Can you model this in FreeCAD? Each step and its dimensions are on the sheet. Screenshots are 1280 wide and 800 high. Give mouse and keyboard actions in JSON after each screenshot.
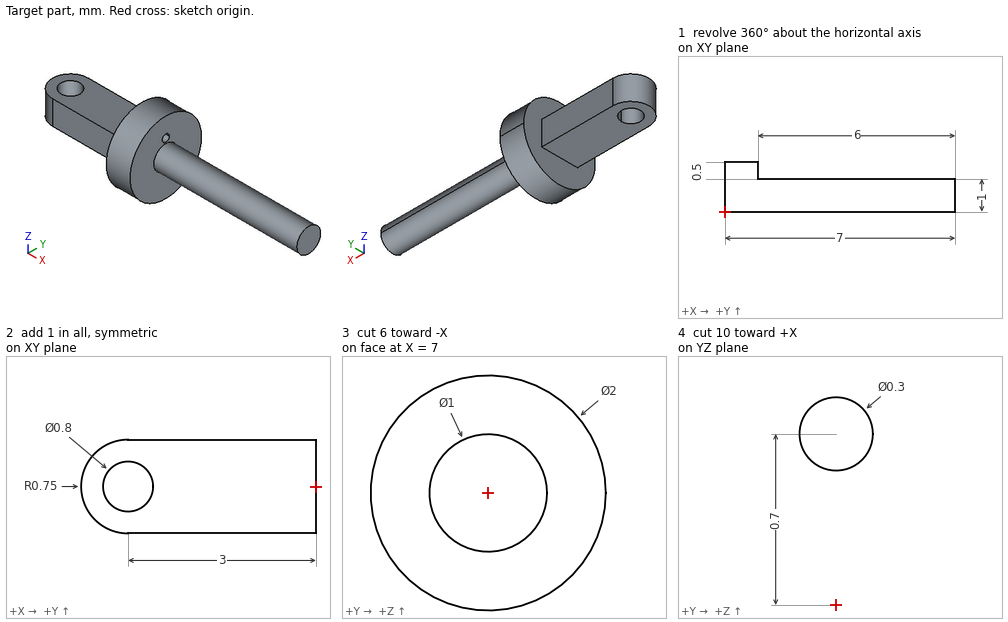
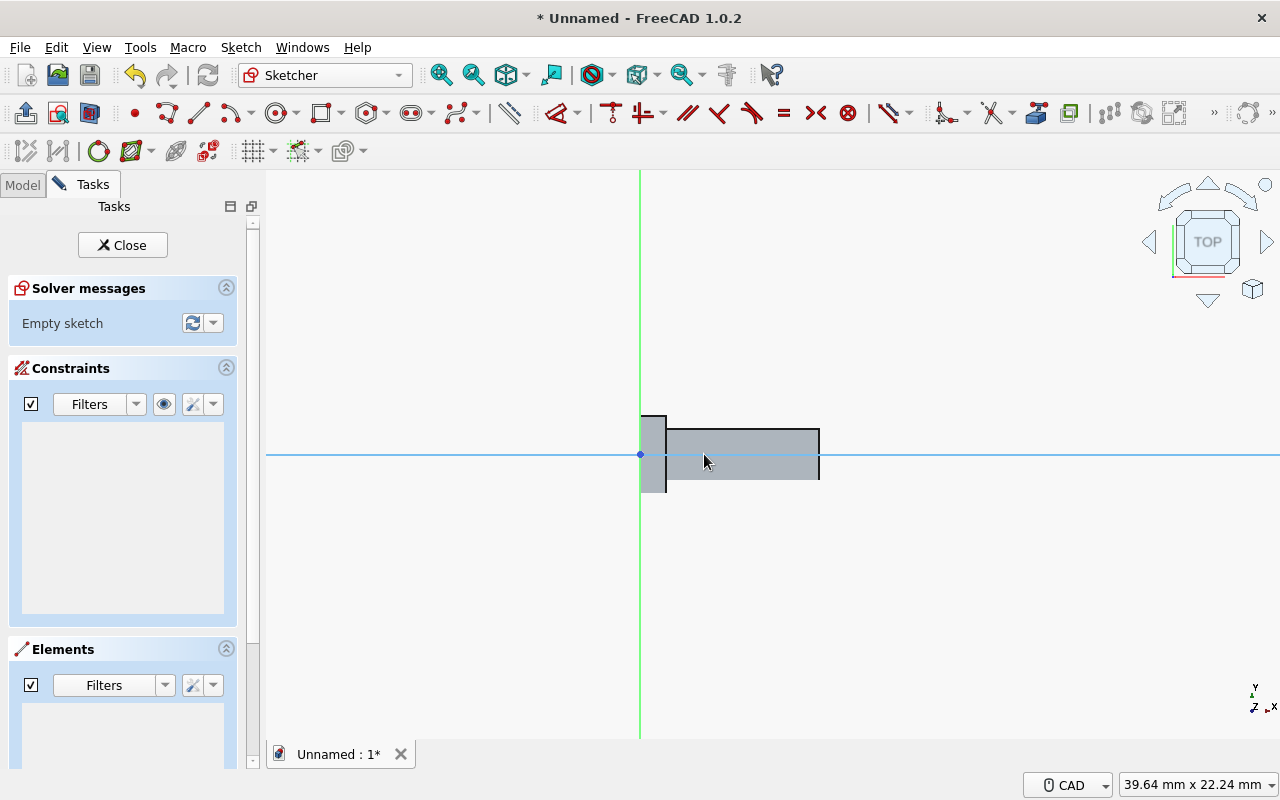
{"action": "scroll", "coordinate": [570, 455], "scroll_direction": "up", "scroll_amount": 9}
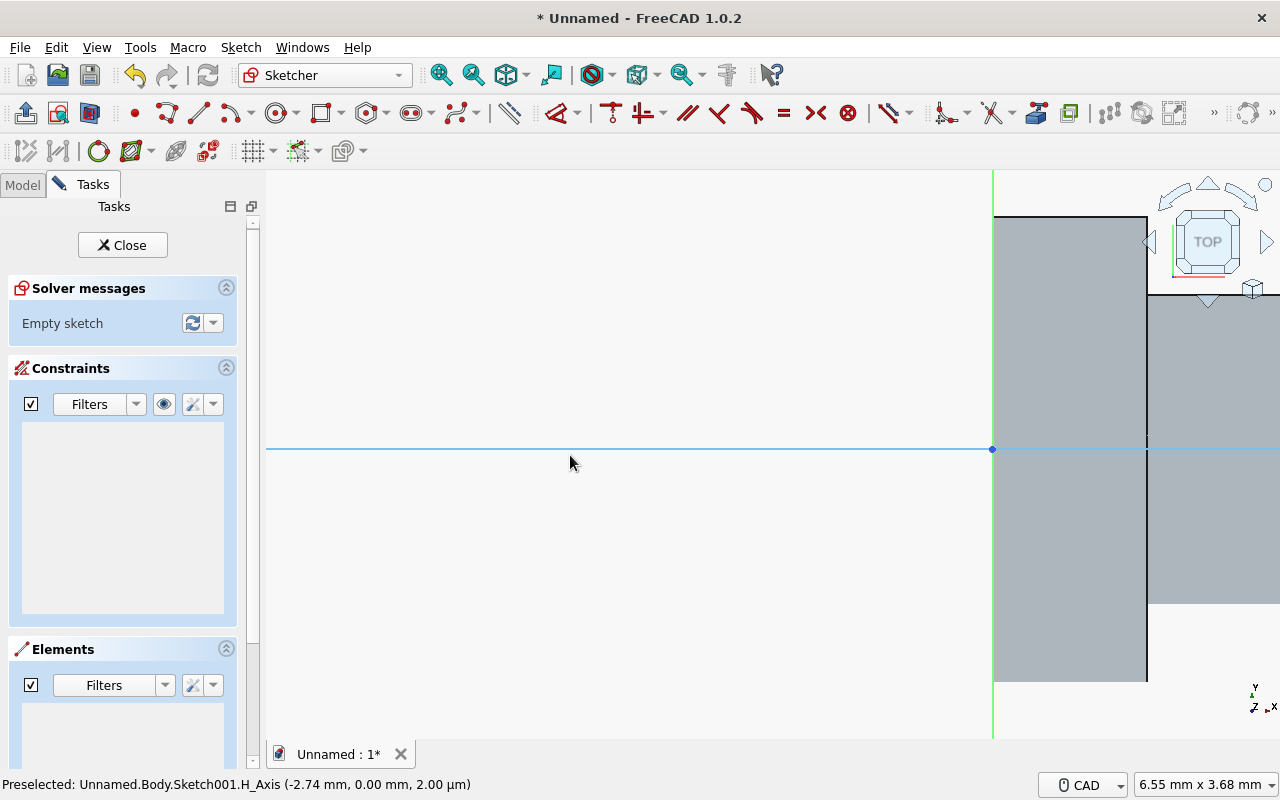
{"action": "left_click", "coordinate": [168, 114]}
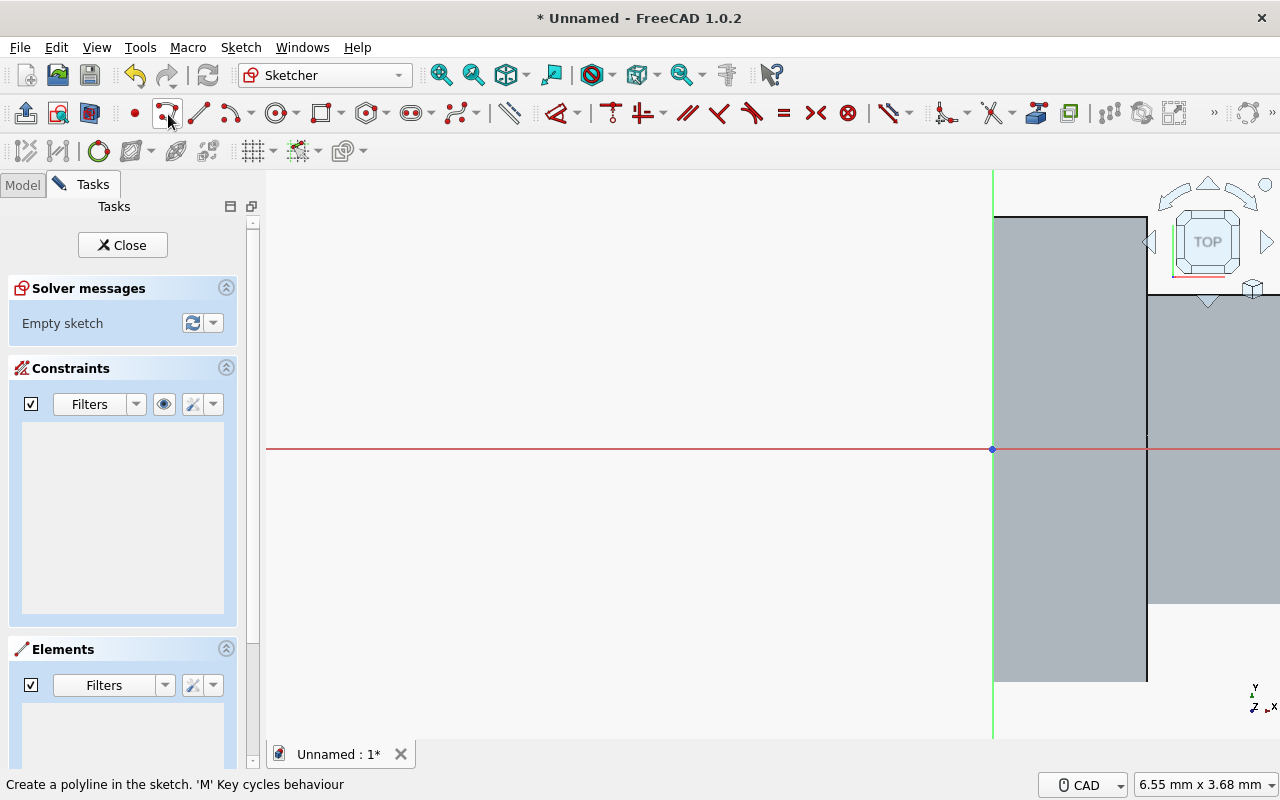
{"action": "left_click", "coordinate": [528, 566]}
{"action": "left_click", "coordinate": [993, 566]}
{"action": "left_click", "coordinate": [984, 333]}
{"action": "left_click", "coordinate": [528, 333]}
{"action": "right_click", "coordinate": [528, 333]}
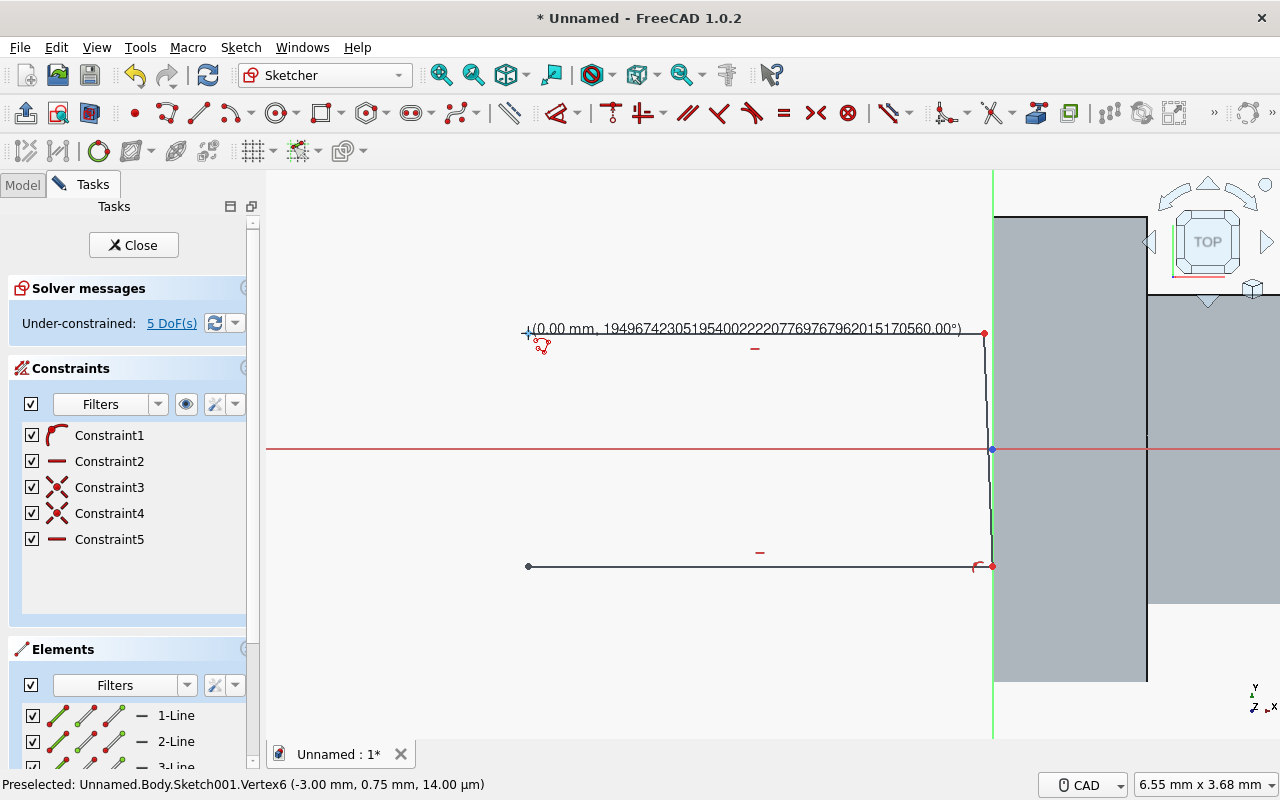
{"action": "left_click", "coordinate": [254, 114]}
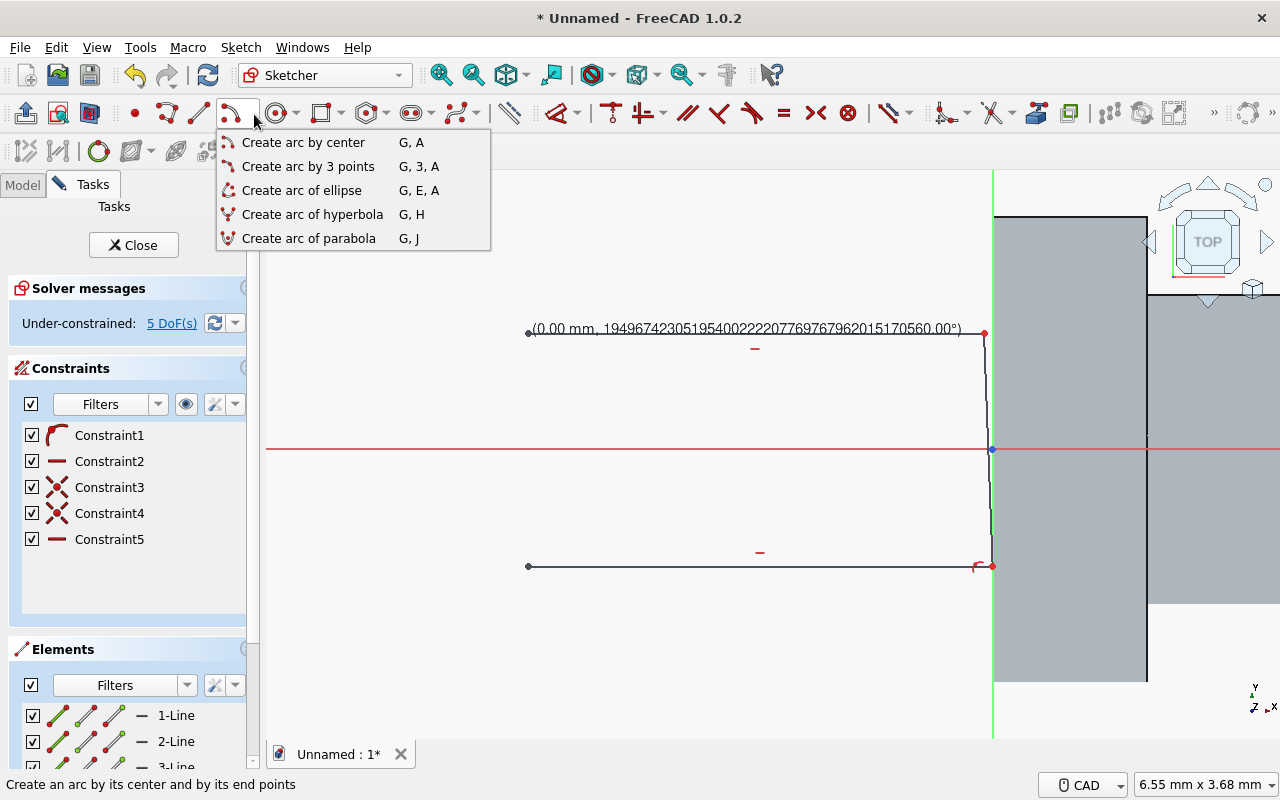
{"action": "left_click", "coordinate": [354, 166]}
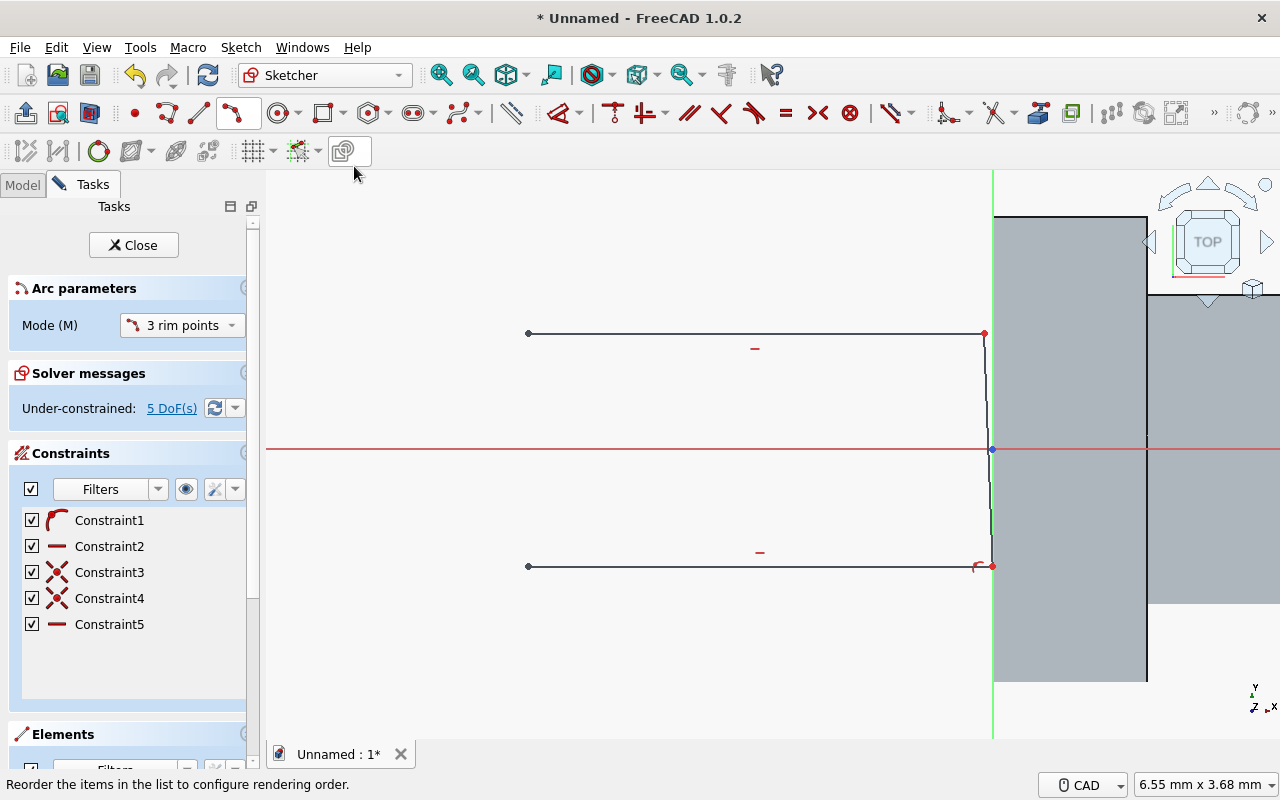
{"action": "left_click", "coordinate": [528, 334]}
{"action": "left_click", "coordinate": [528, 567]}
{"action": "left_click", "coordinate": [418, 414]}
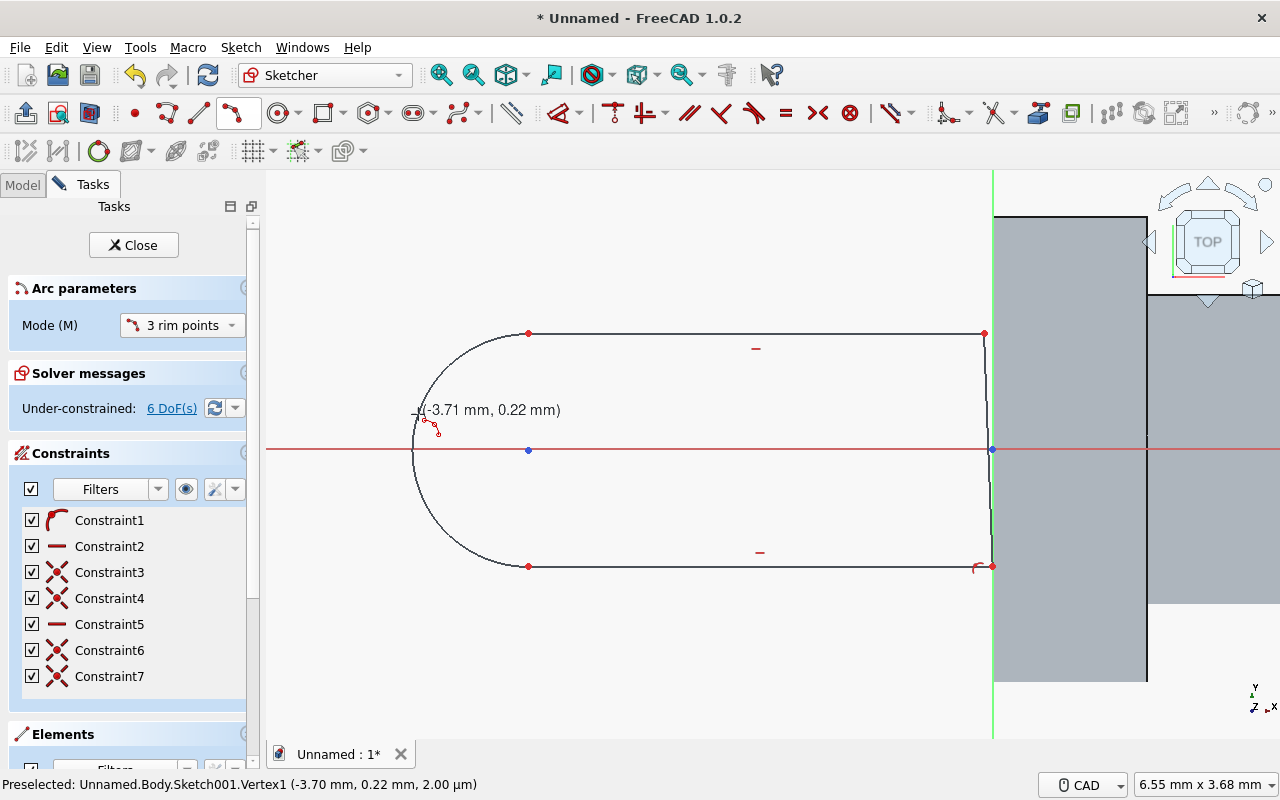
{"action": "left_click", "coordinate": [278, 114]}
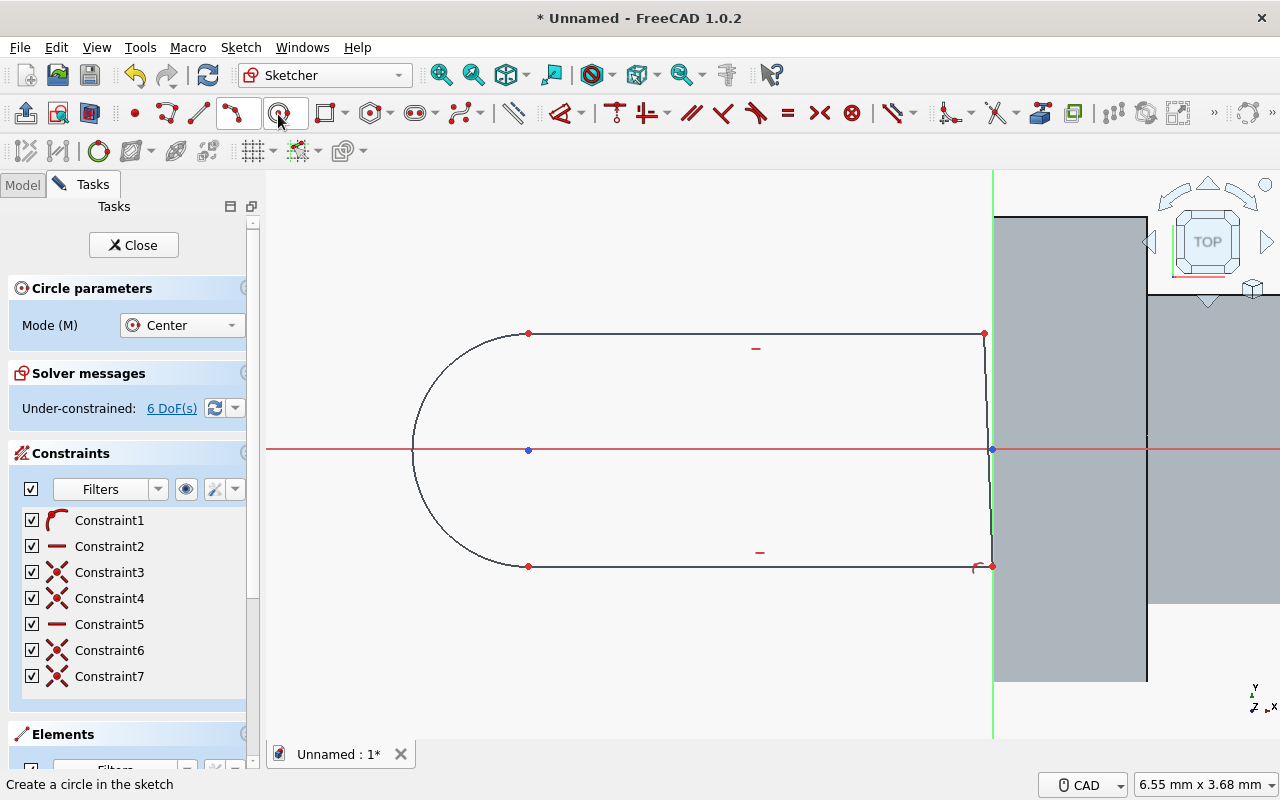
{"action": "left_click", "coordinate": [528, 449]}
{"action": "left_click", "coordinate": [572, 406]}
{"action": "key", "text": "Escape"}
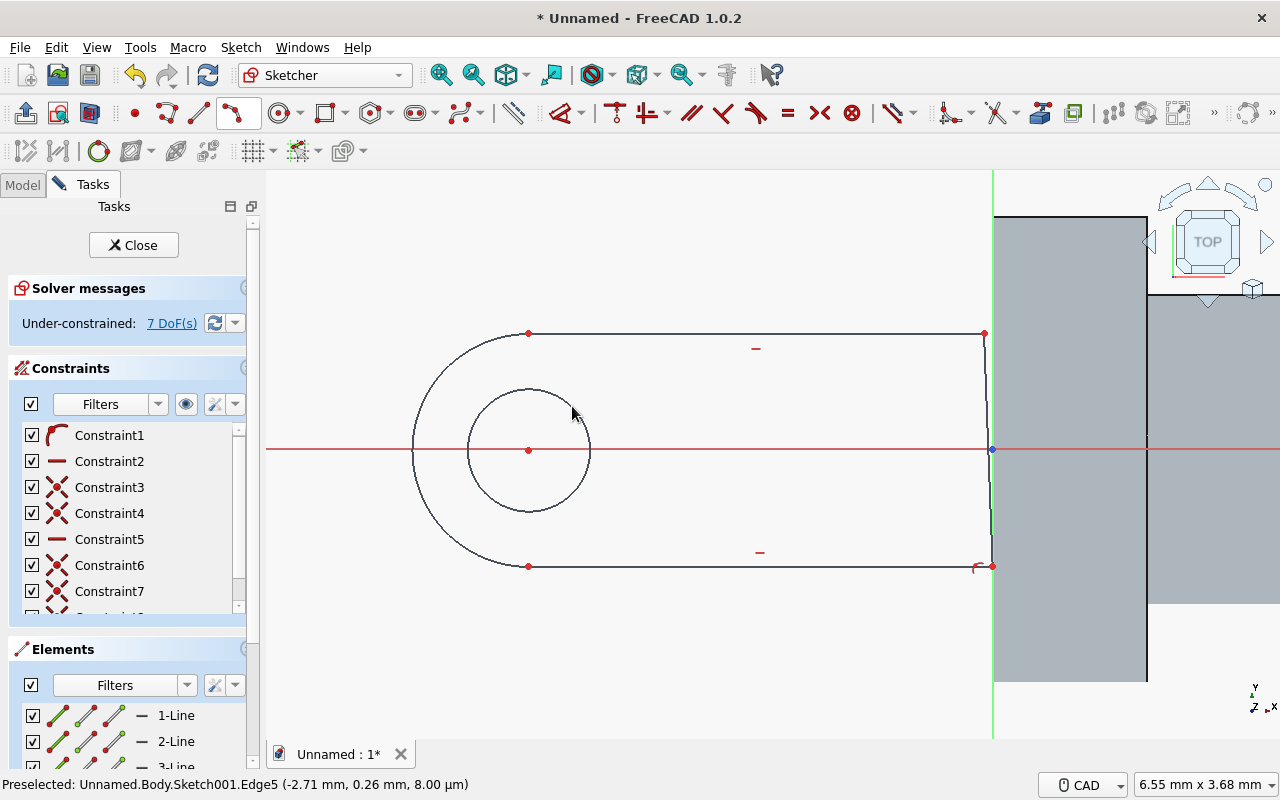
{"action": "left_click", "coordinate": [667, 567]}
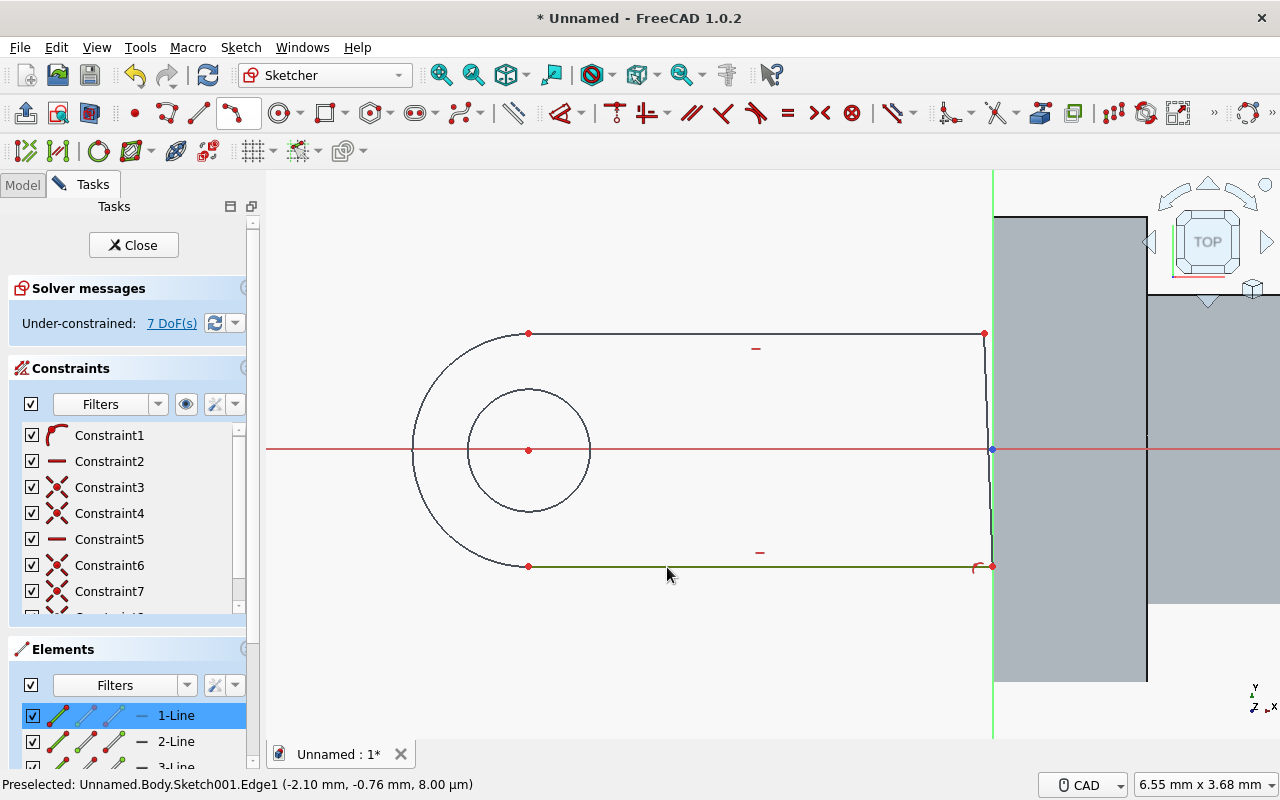
{"action": "left_click", "coordinate": [434, 382]}